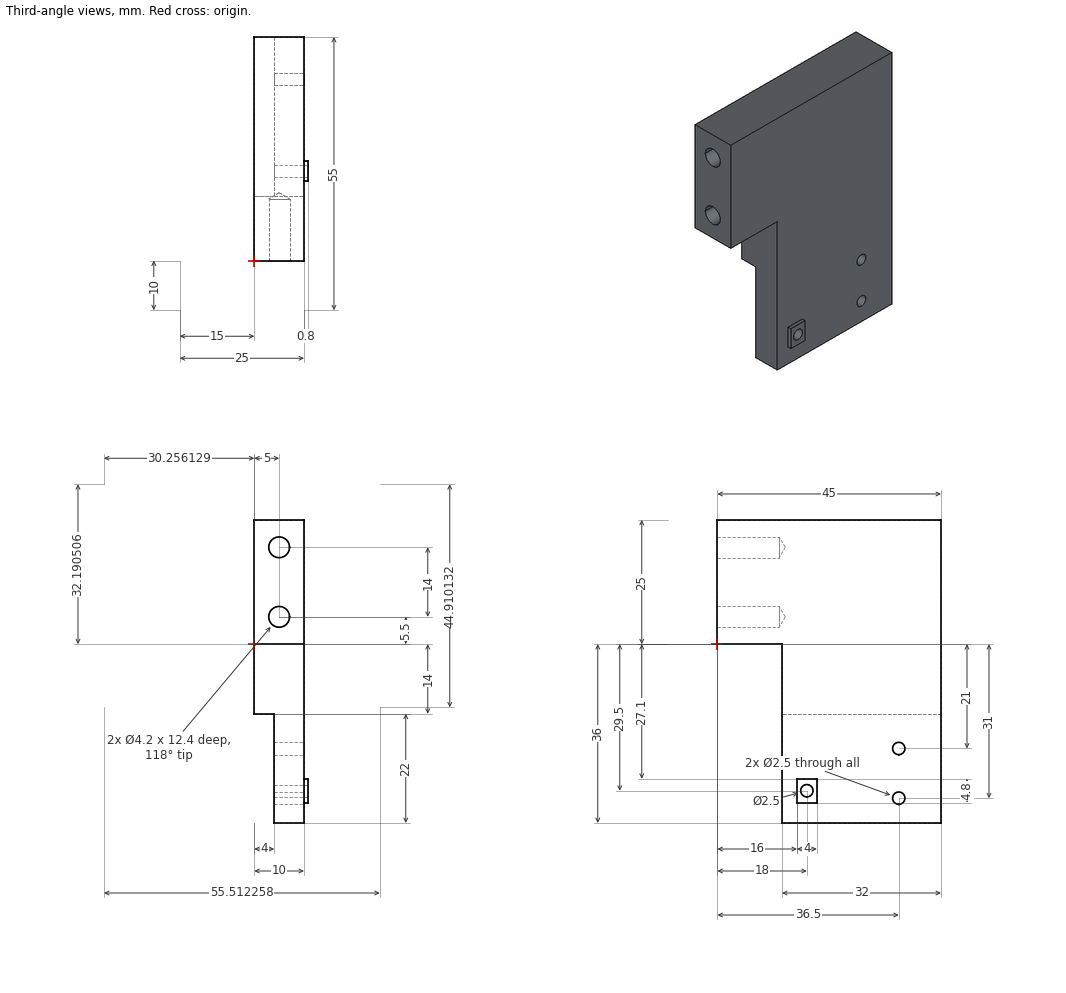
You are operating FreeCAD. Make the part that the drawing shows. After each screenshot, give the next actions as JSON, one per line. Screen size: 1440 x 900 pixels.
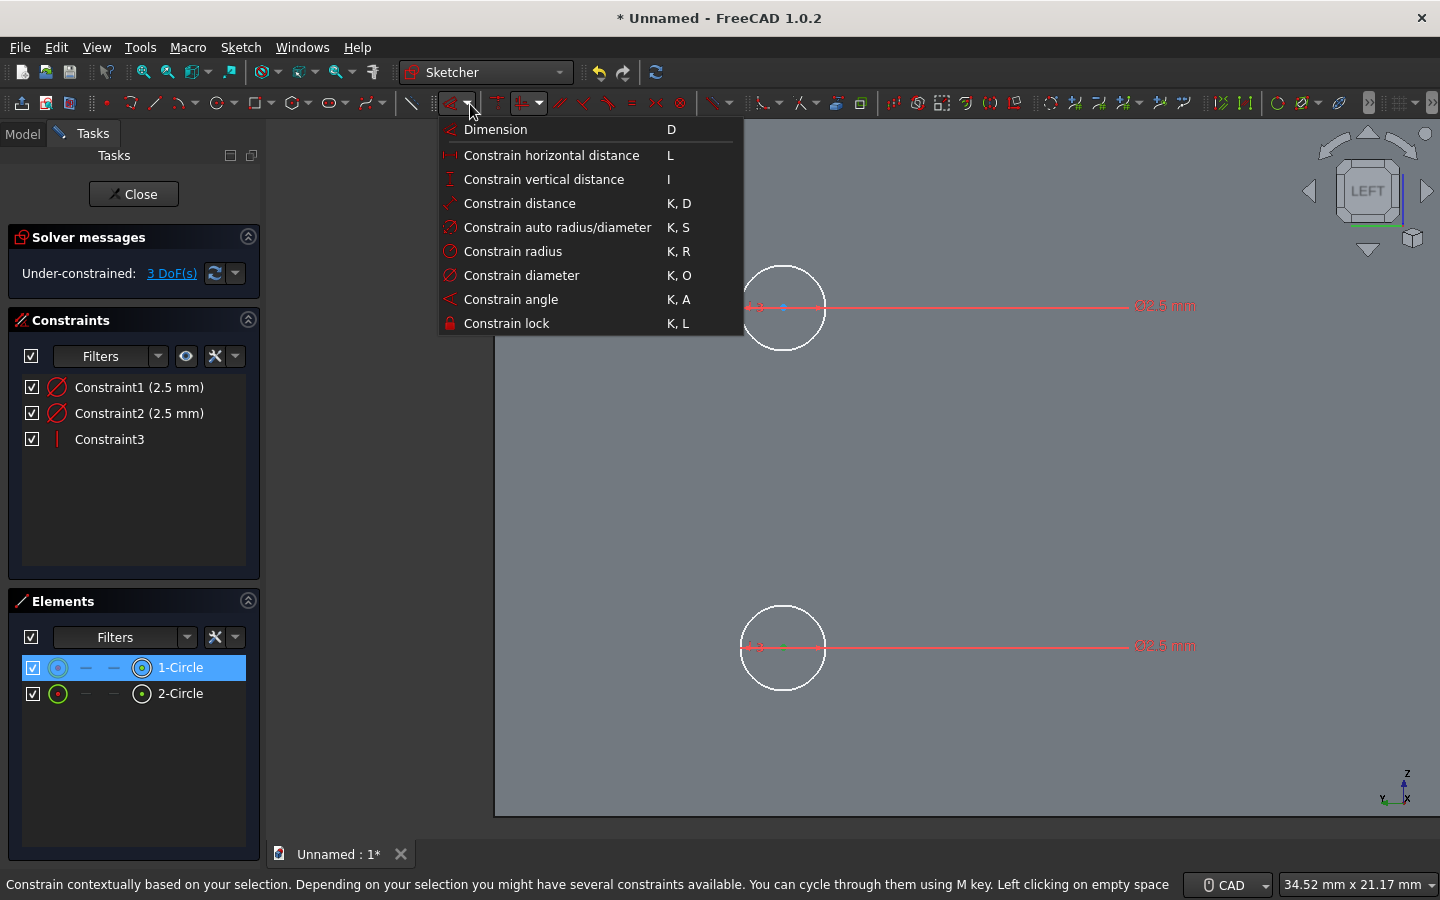
{"action": "left_click", "coordinate": [591, 179]}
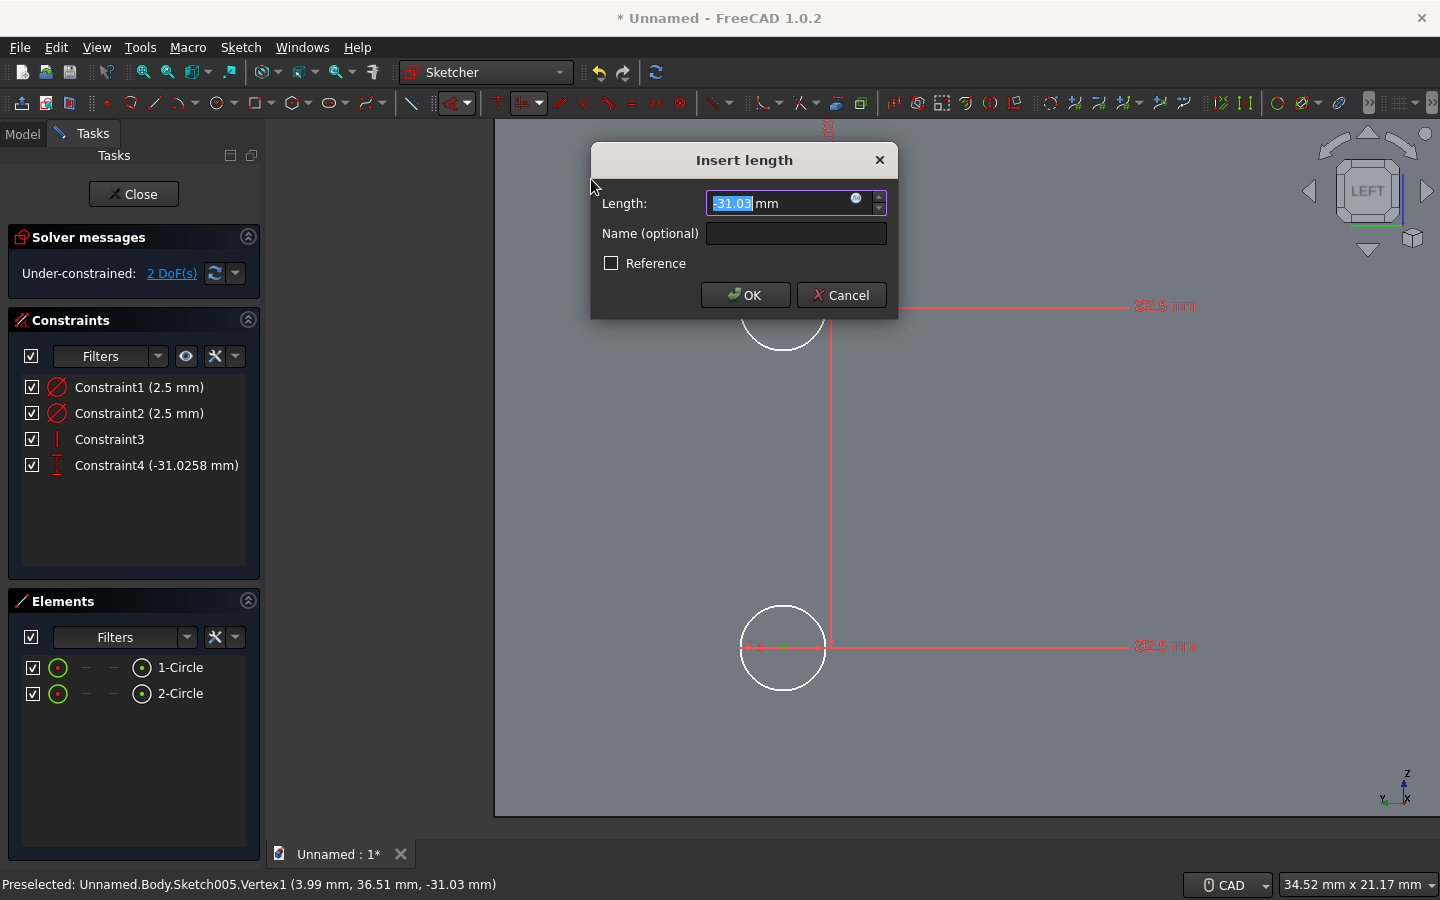
{"action": "type", "text": "-31"}
{"action": "key", "text": "Return"}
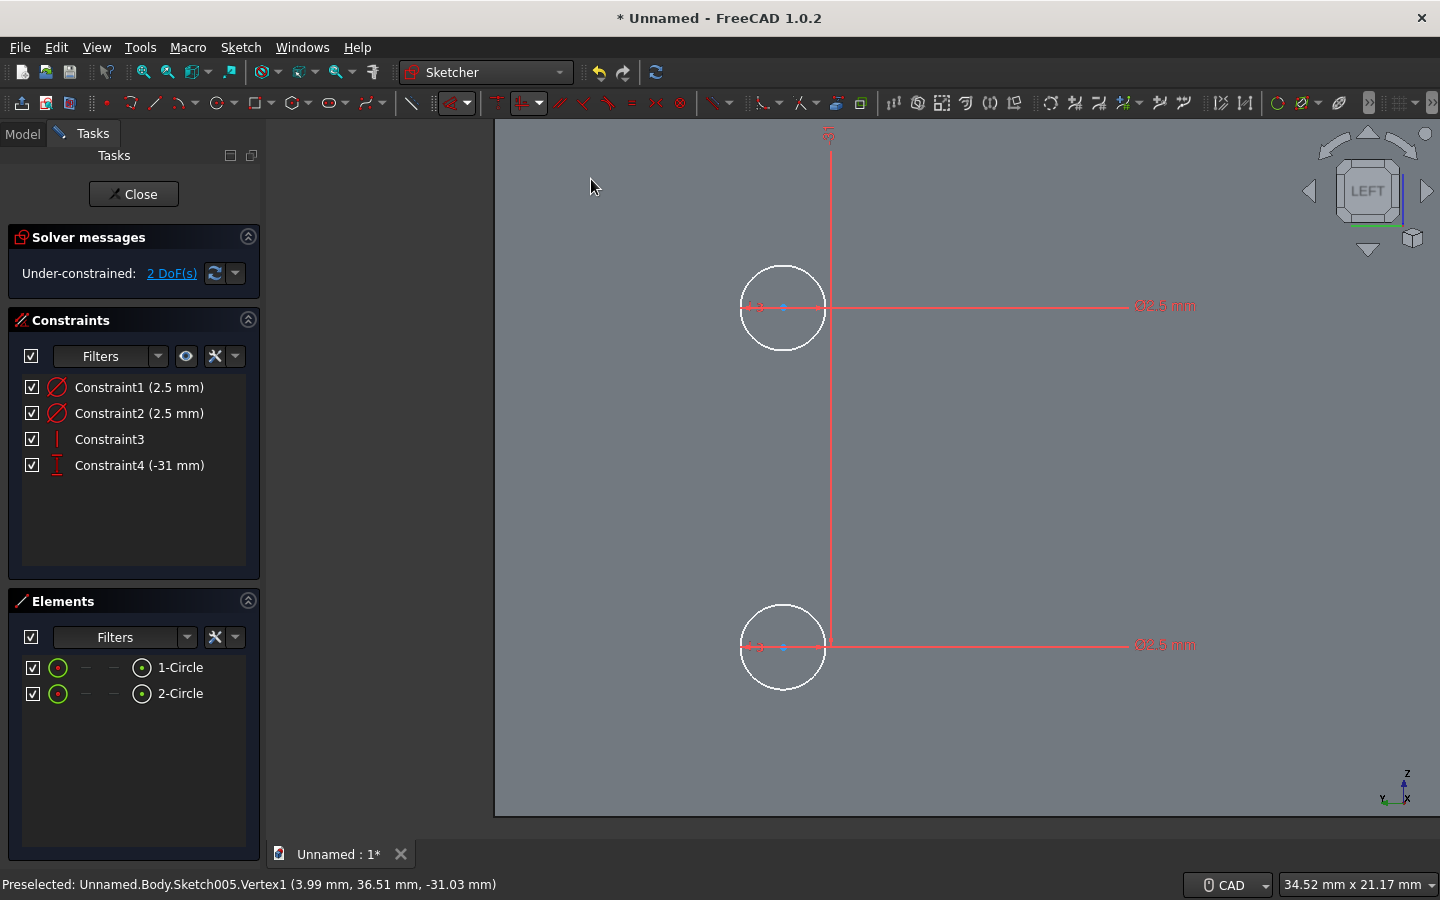
{"action": "left_click", "coordinate": [783, 308]}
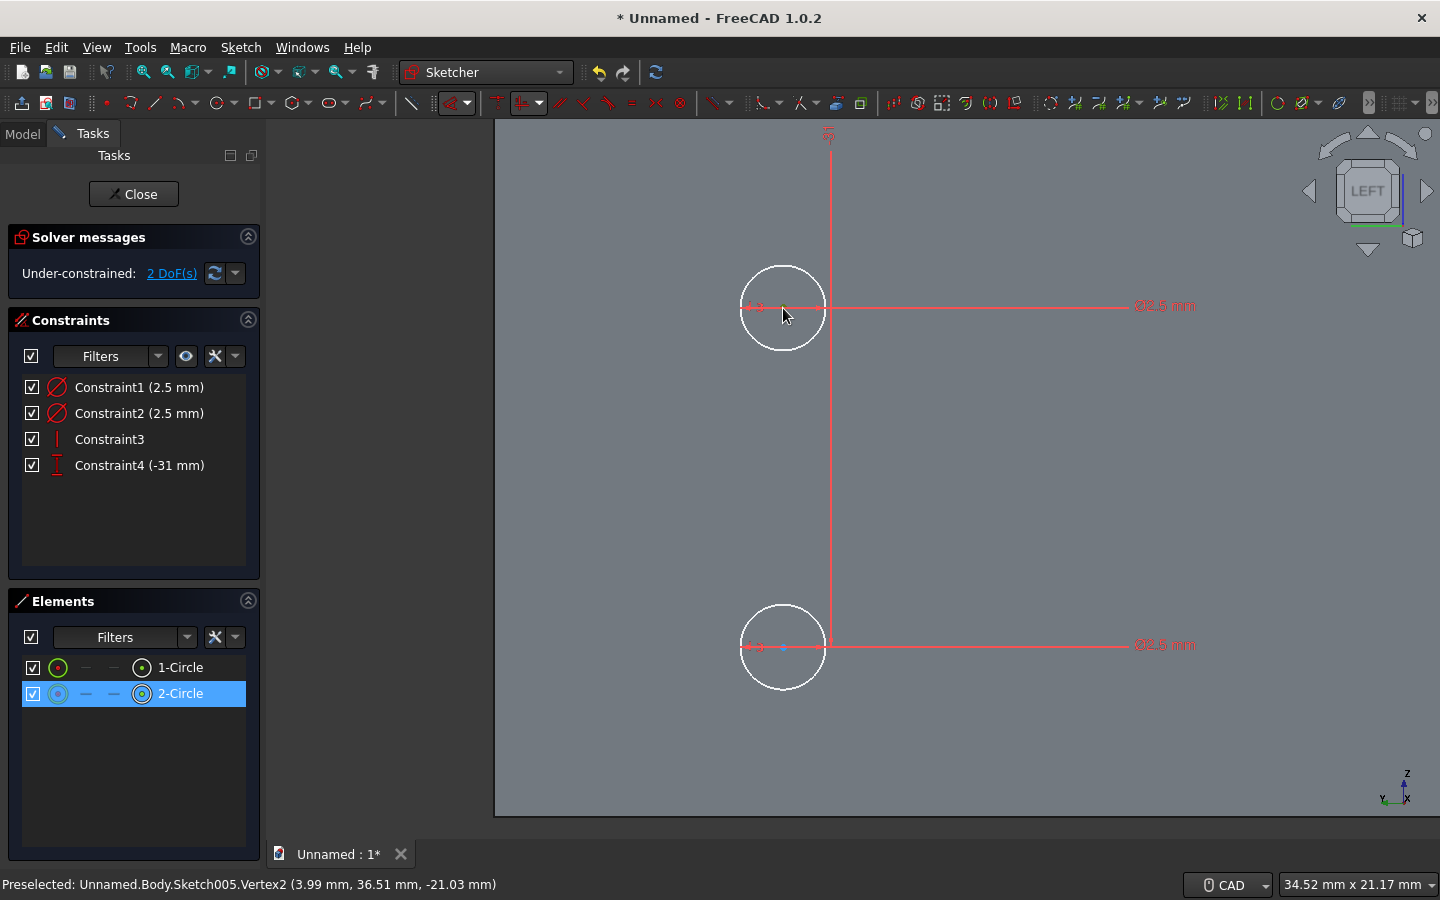
{"action": "key", "text": "i"}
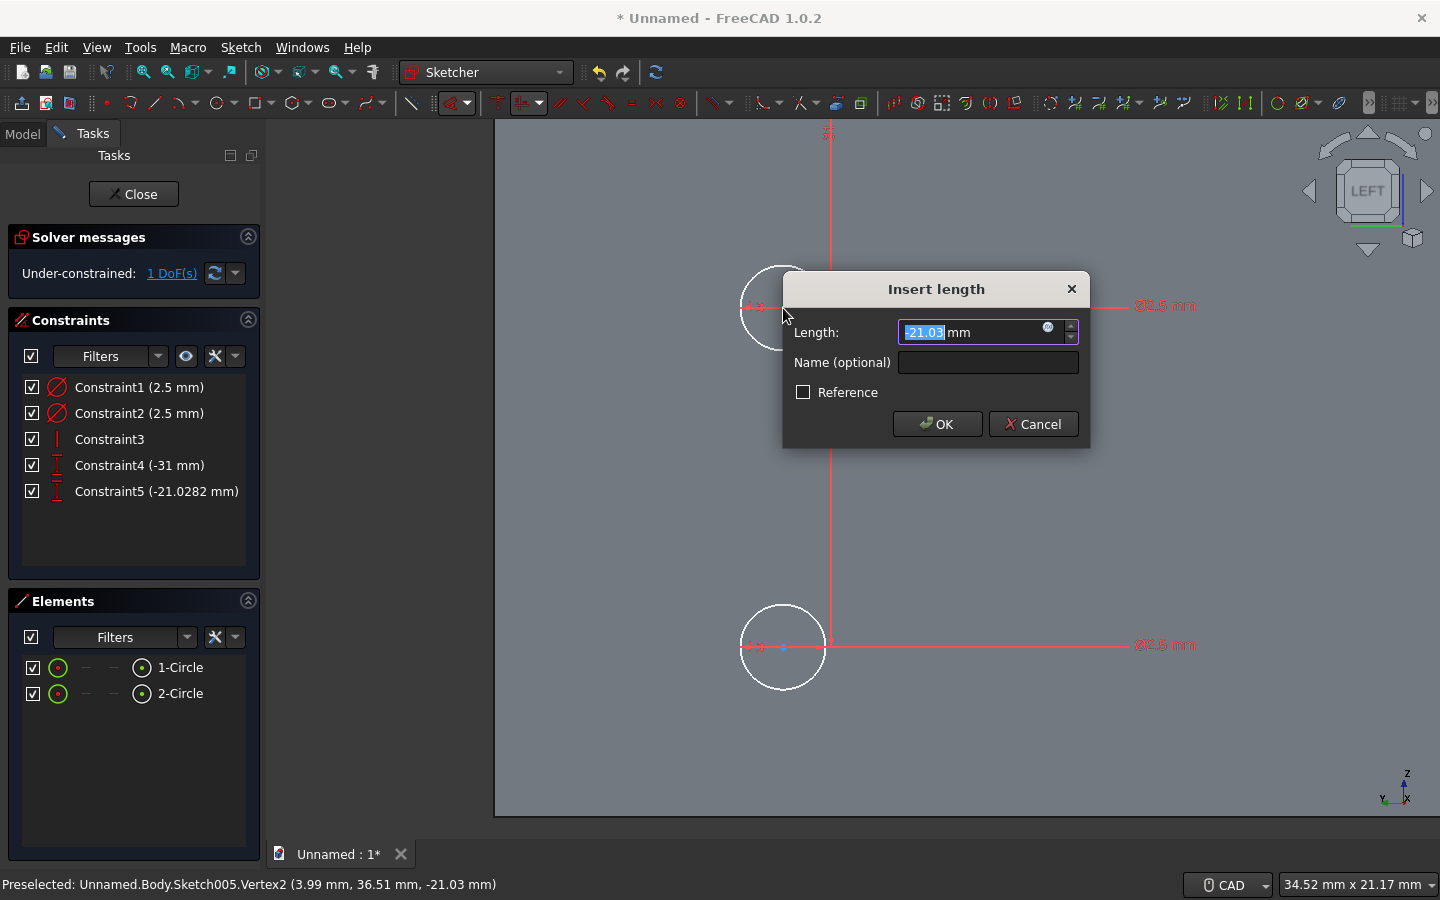
{"action": "type", "text": "-21"}
{"action": "key", "text": "Return"}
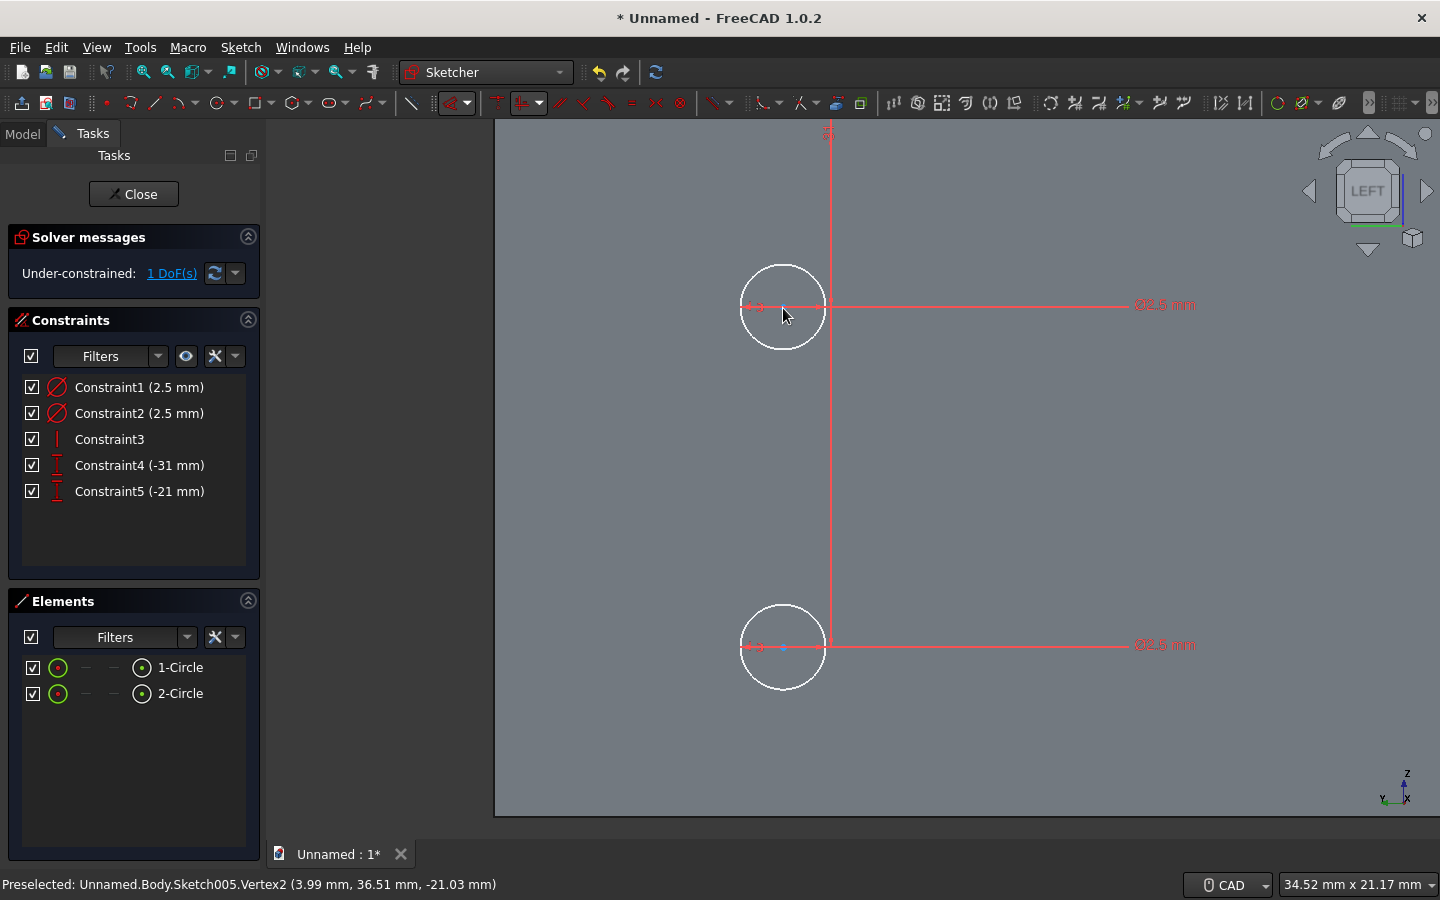
{"action": "left_click", "coordinate": [783, 647]}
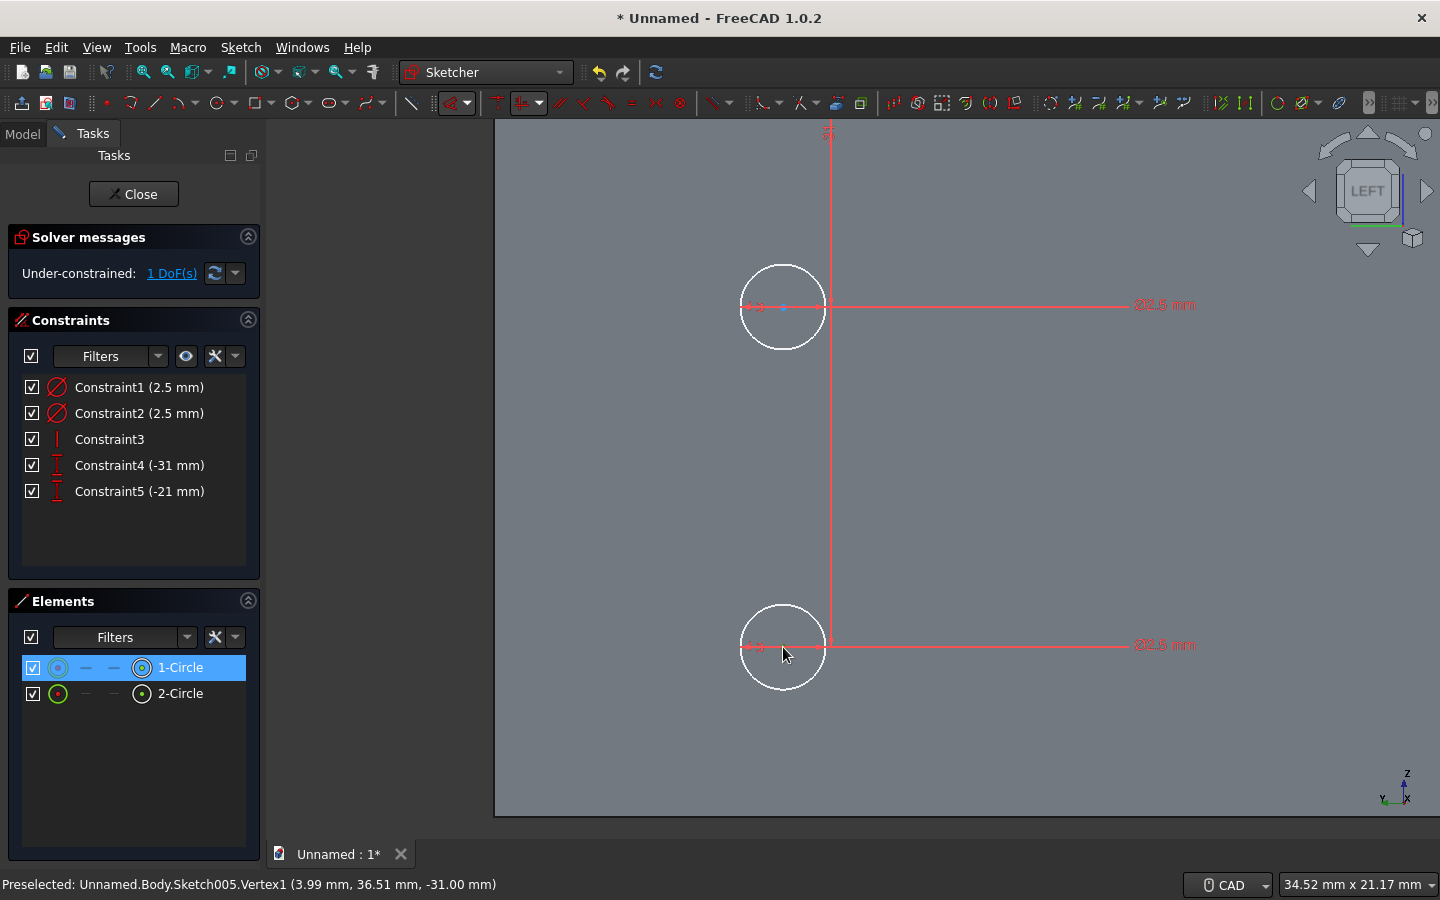
{"action": "key", "text": "l"}